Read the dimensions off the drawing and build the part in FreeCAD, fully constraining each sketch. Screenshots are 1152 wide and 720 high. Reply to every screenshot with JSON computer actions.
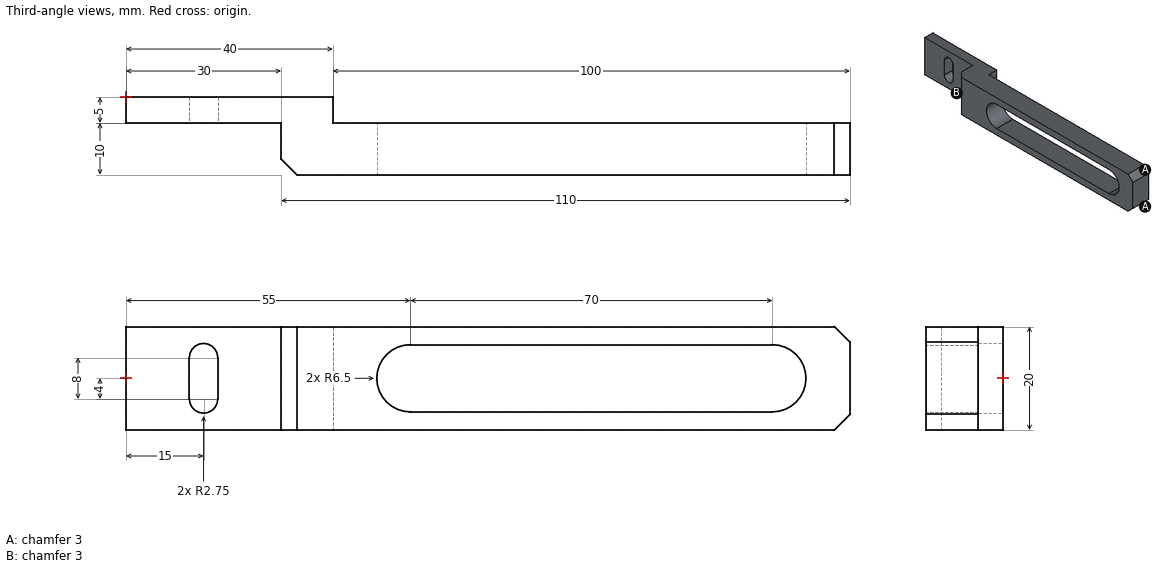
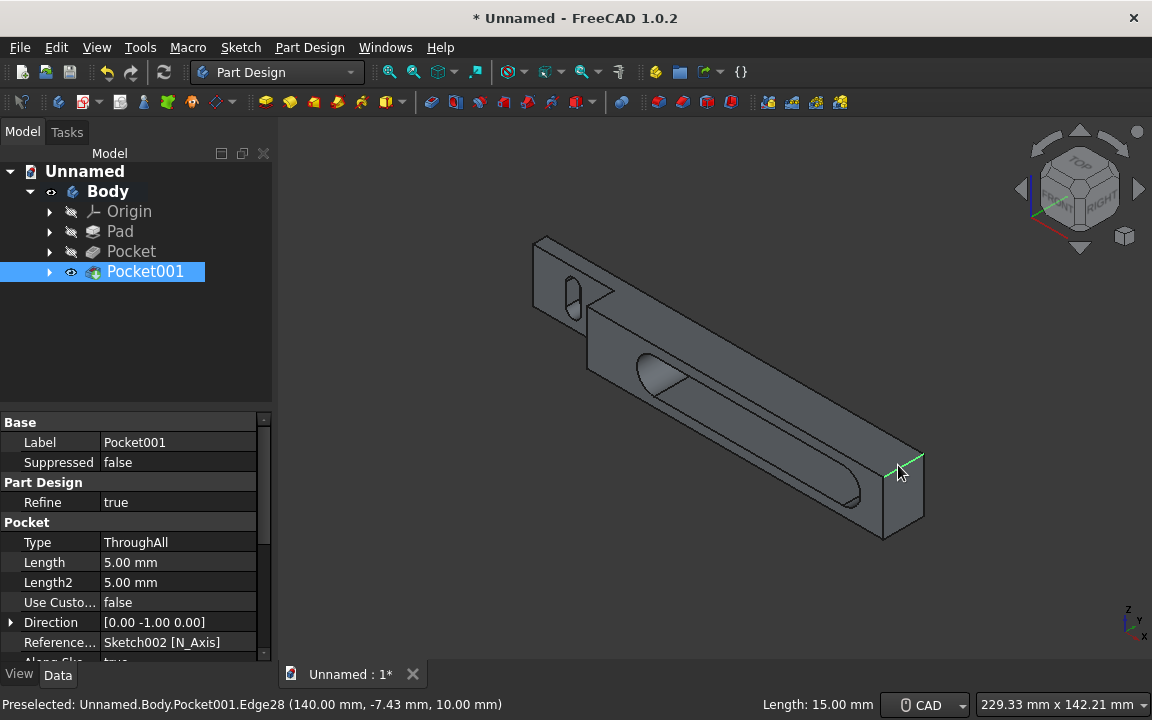
{"action": "key", "text": "2"}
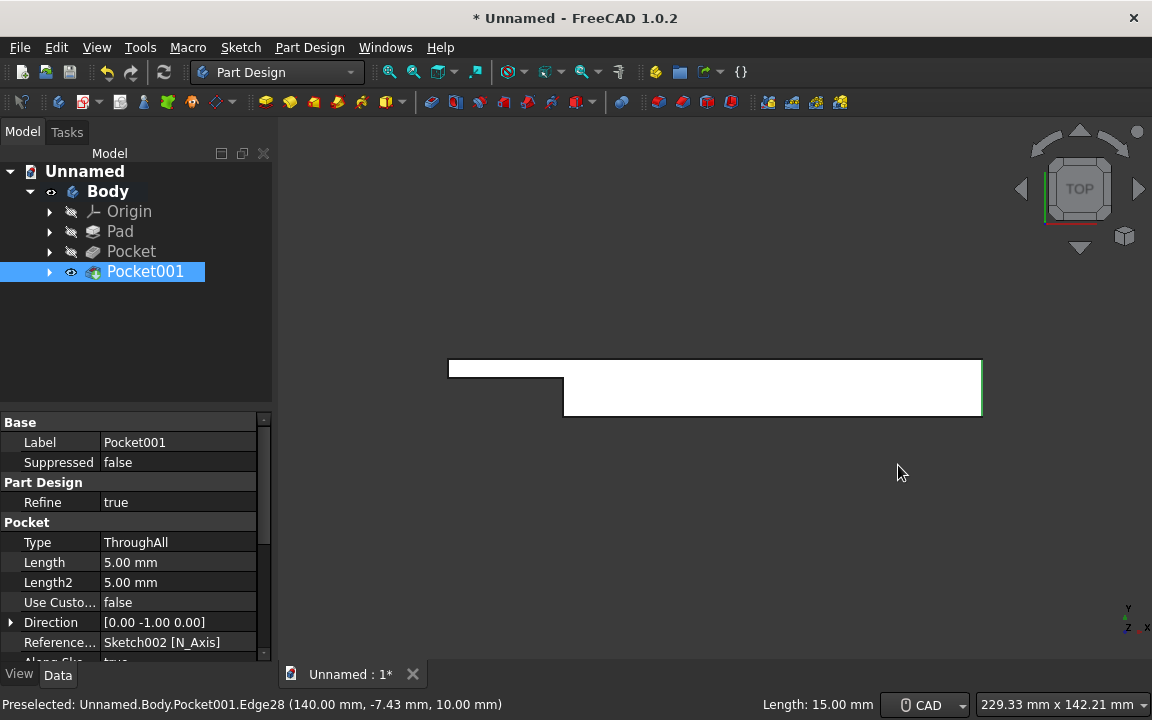
{"action": "key", "text": "1"}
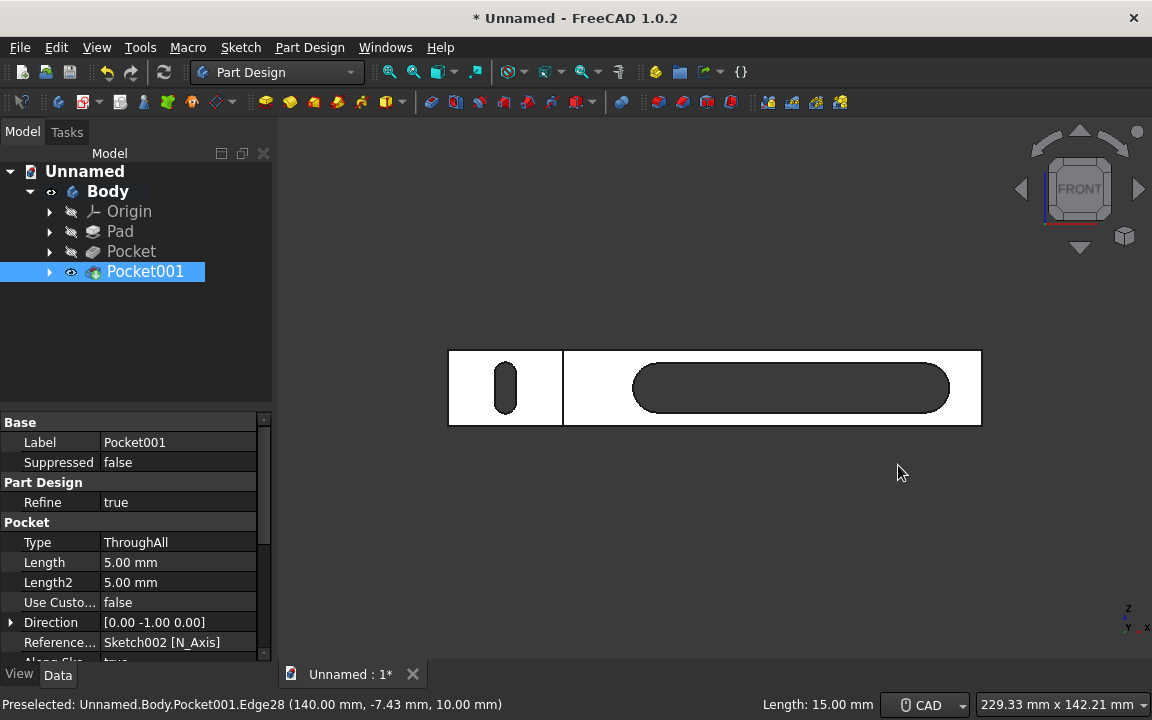
{"action": "key", "text": "3"}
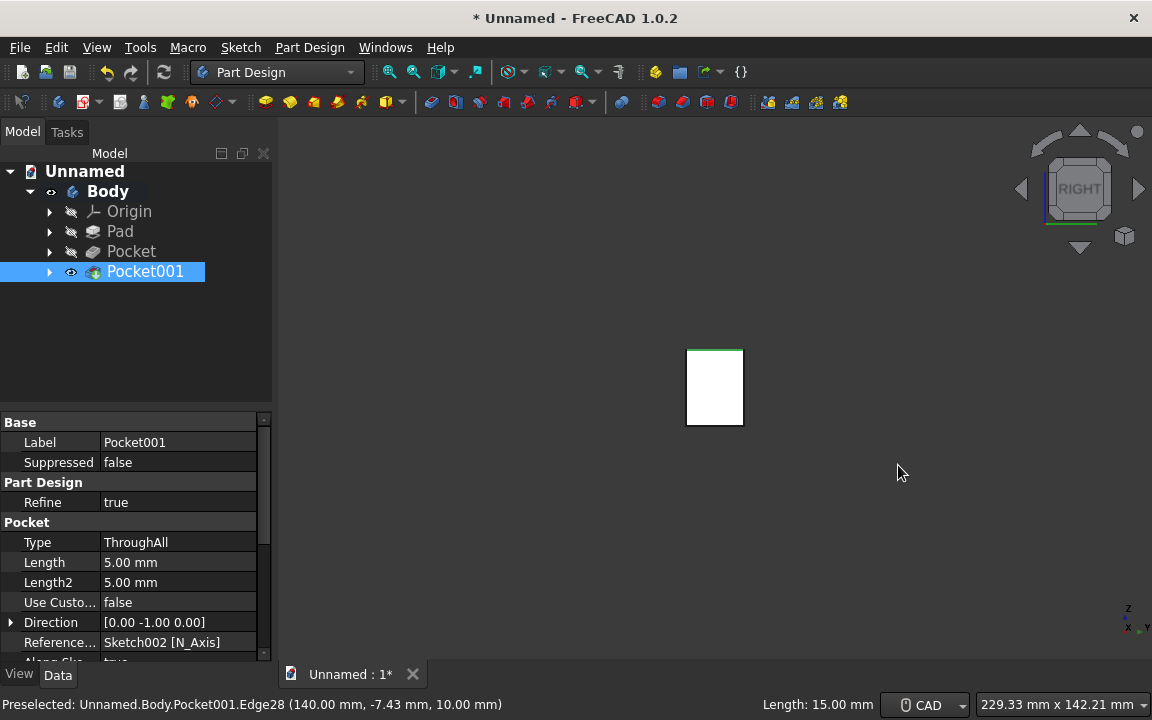
{"action": "left_click", "coordinate": [390, 72]}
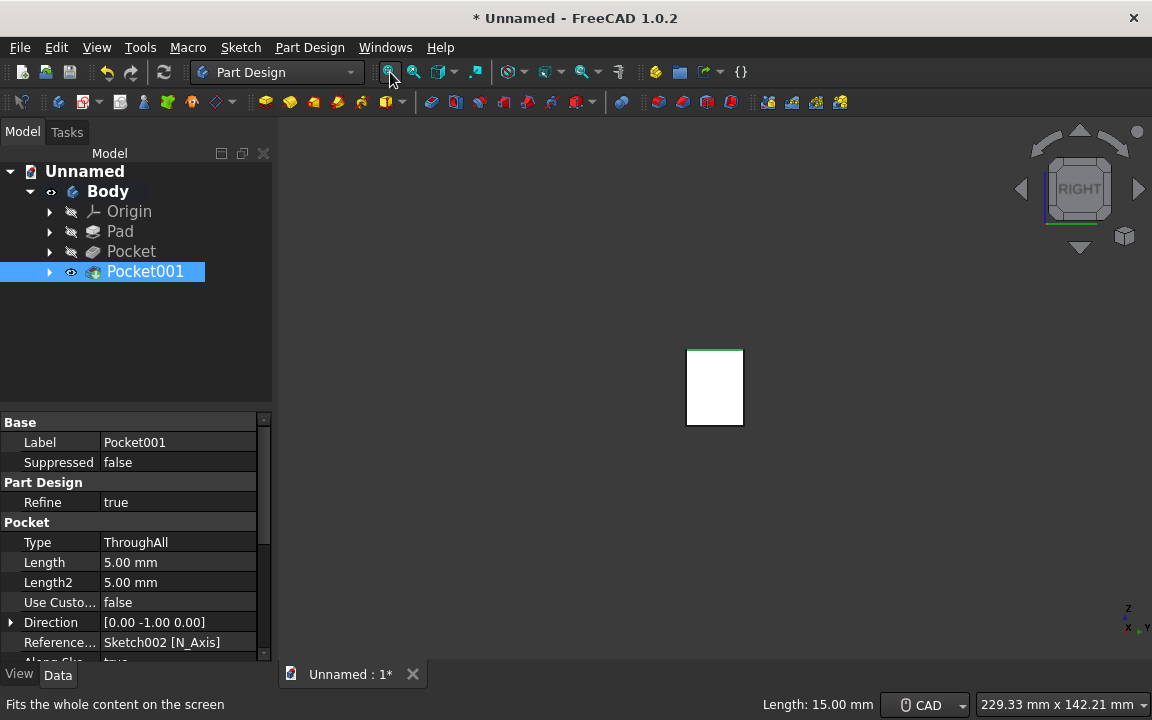
{"action": "left_click", "coordinate": [715, 425], "text": "ctrl"}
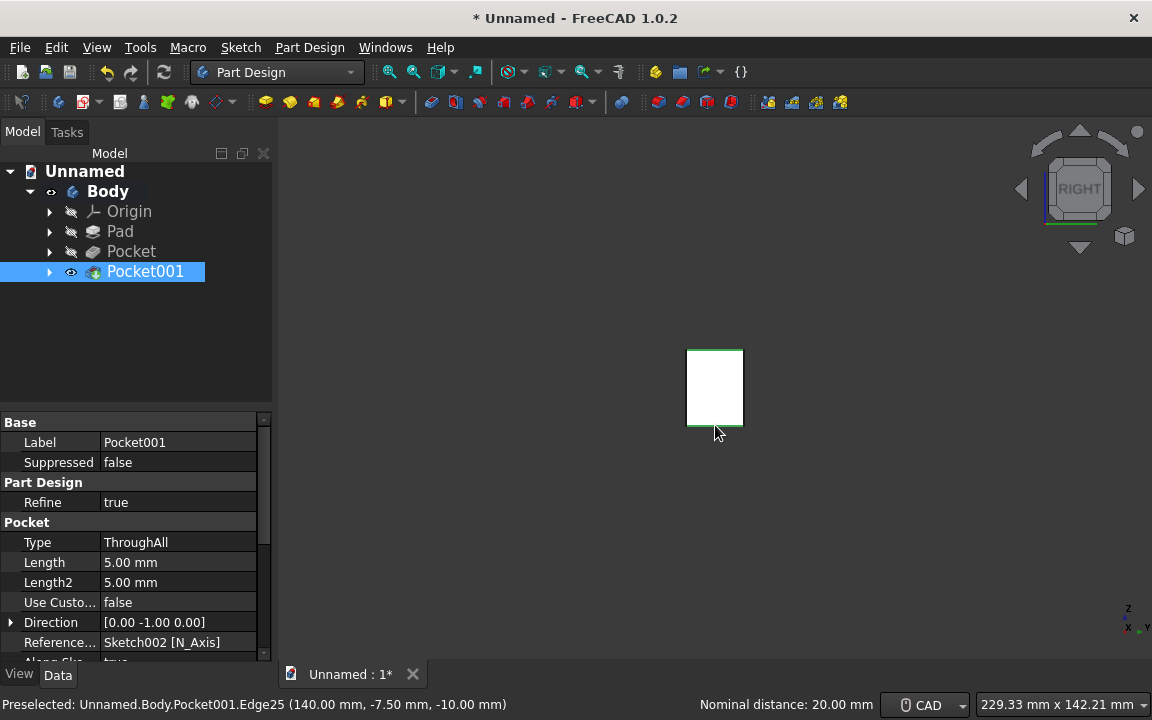
{"action": "left_click", "coordinate": [684, 102]}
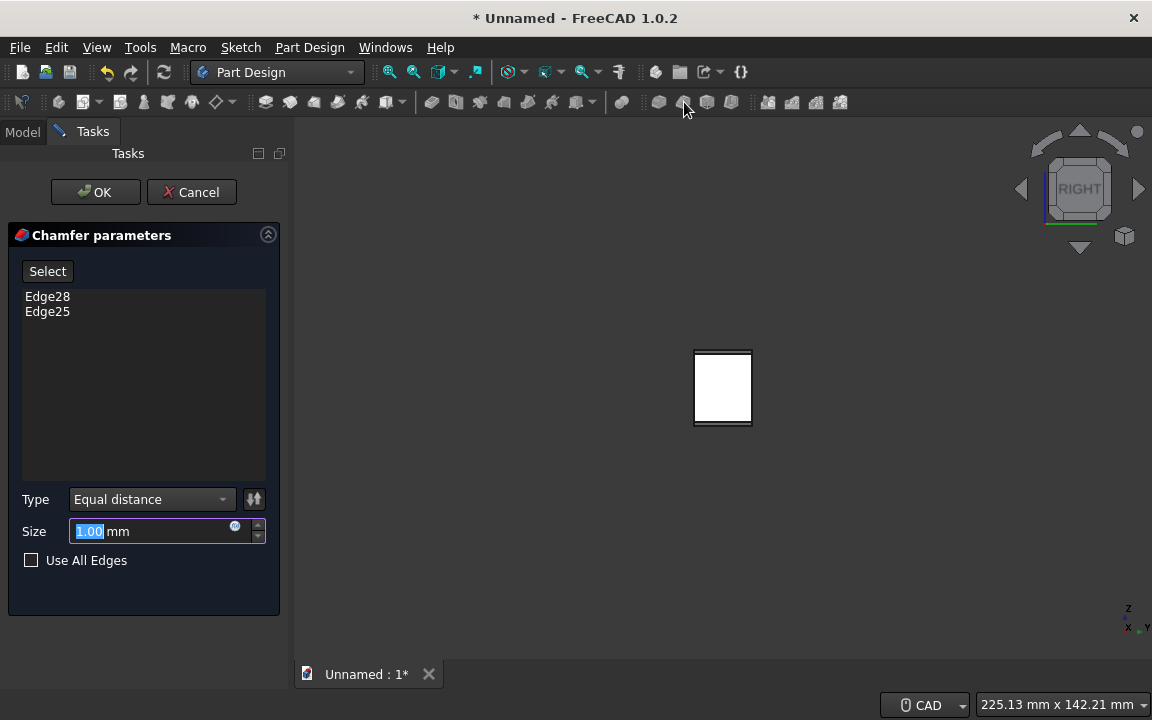
{"action": "type", "text": "3"}
{"action": "key", "text": "Tab"}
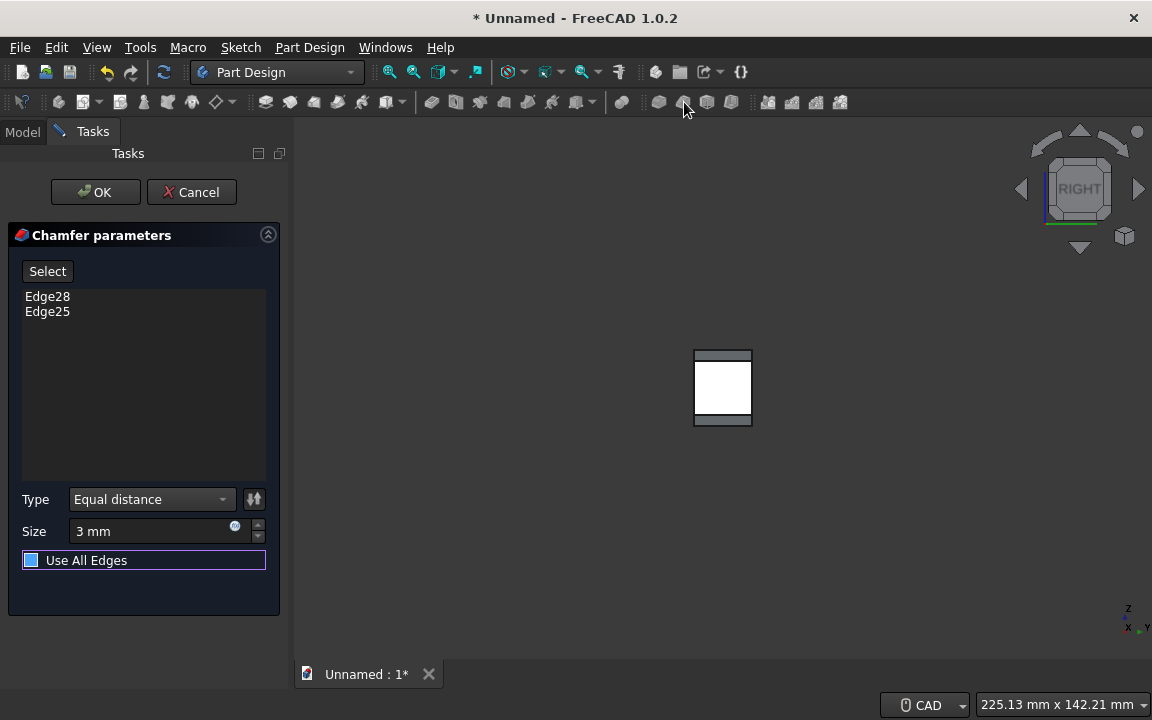
{"action": "left_click", "coordinate": [96, 192]}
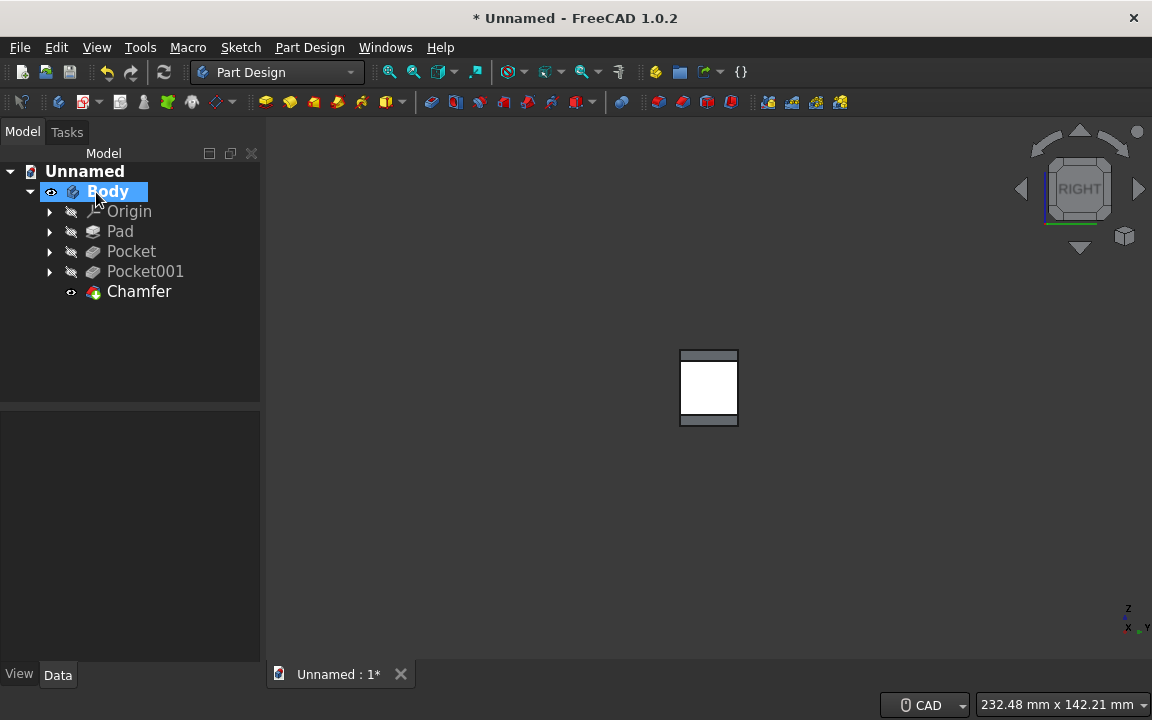
{"action": "key", "text": "v f"}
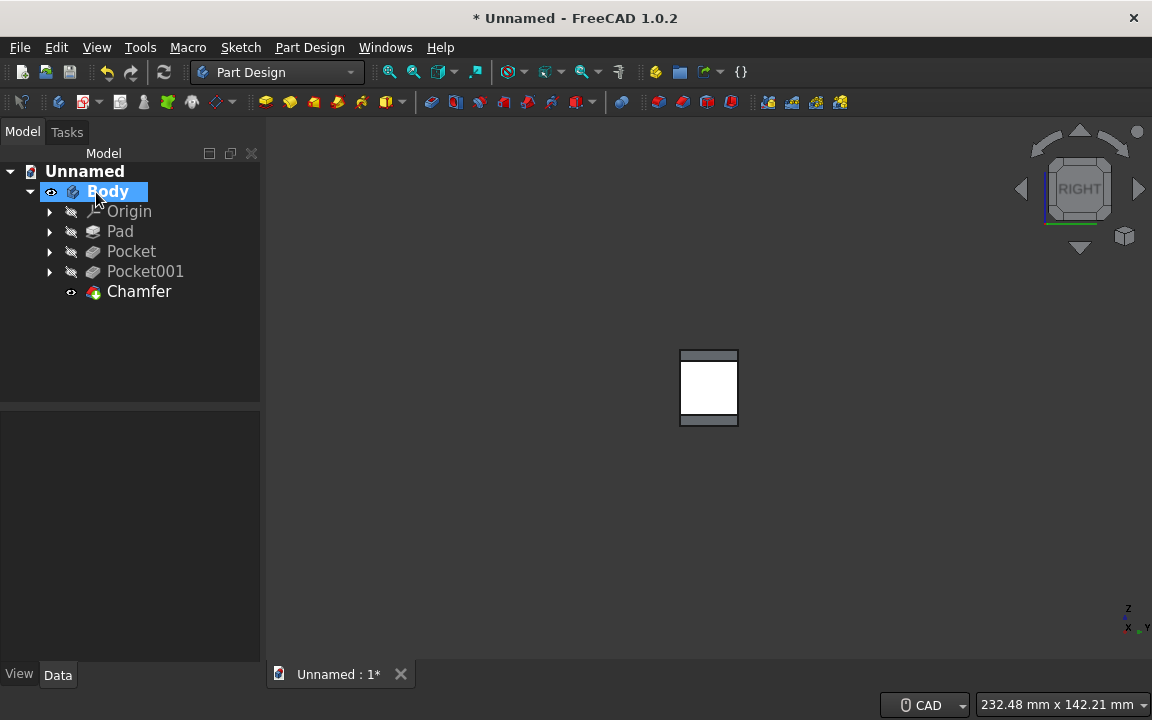
{"action": "key", "text": "0"}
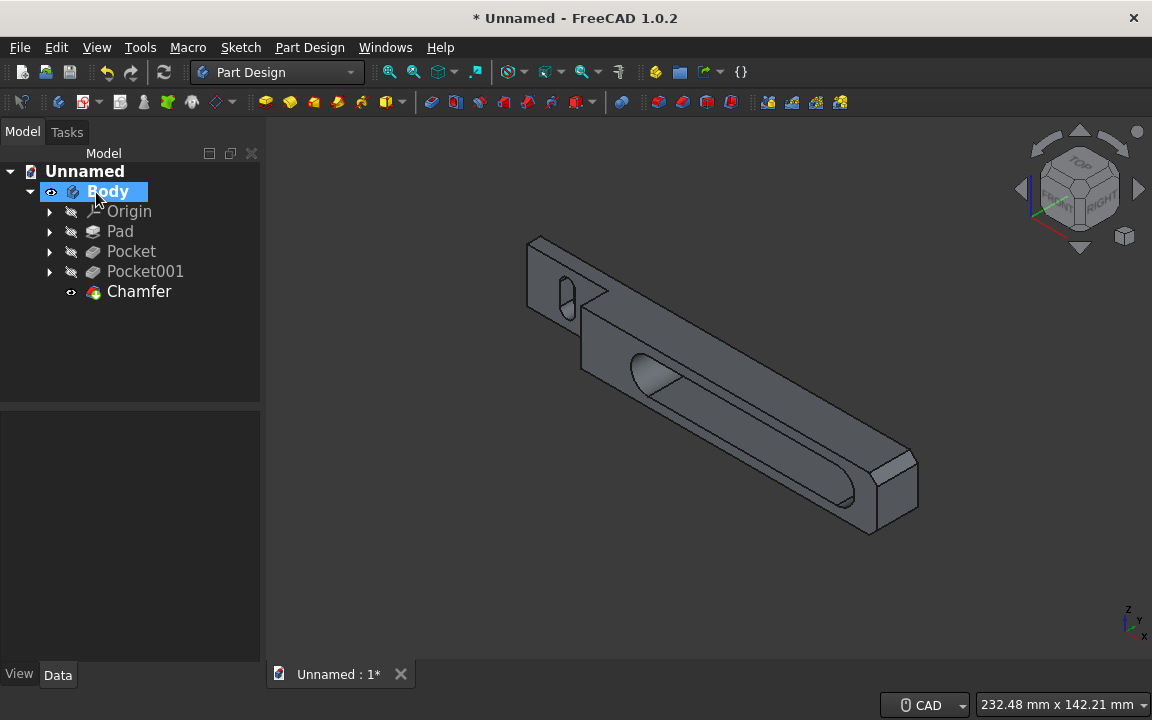
{"action": "key", "text": "2"}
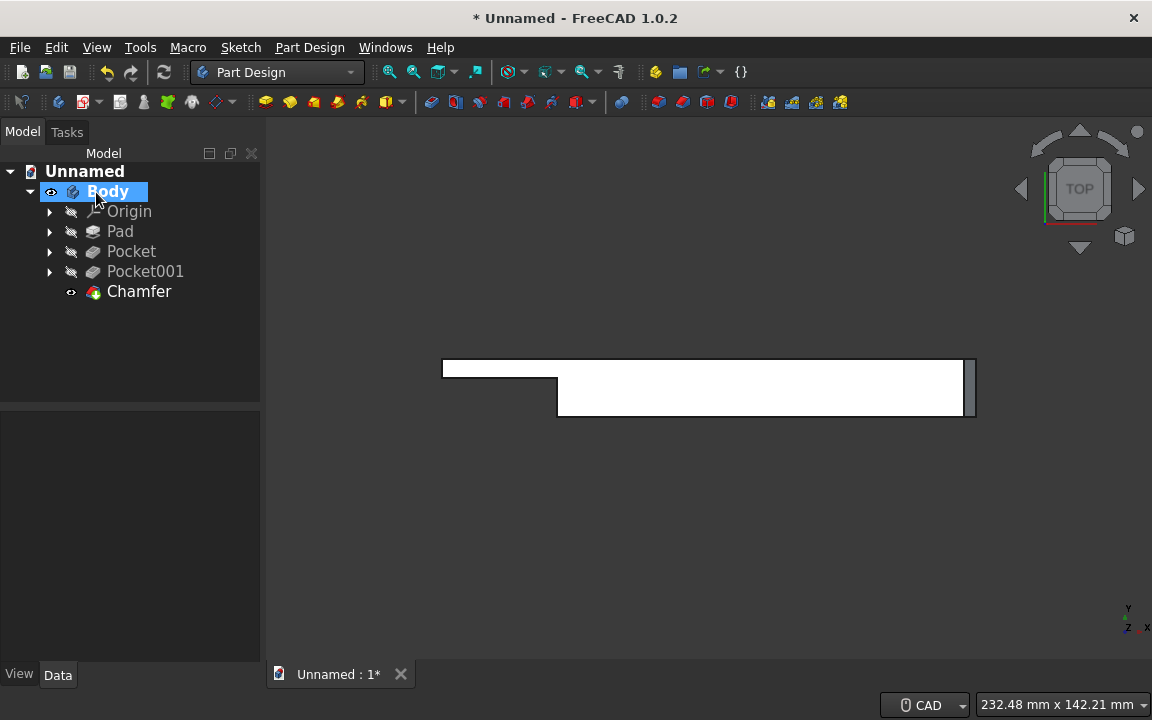
{"action": "key", "text": "1"}